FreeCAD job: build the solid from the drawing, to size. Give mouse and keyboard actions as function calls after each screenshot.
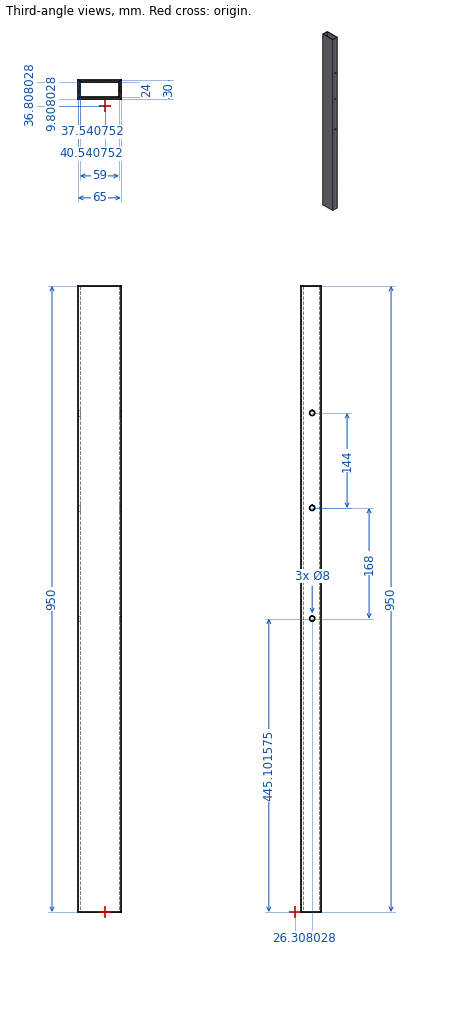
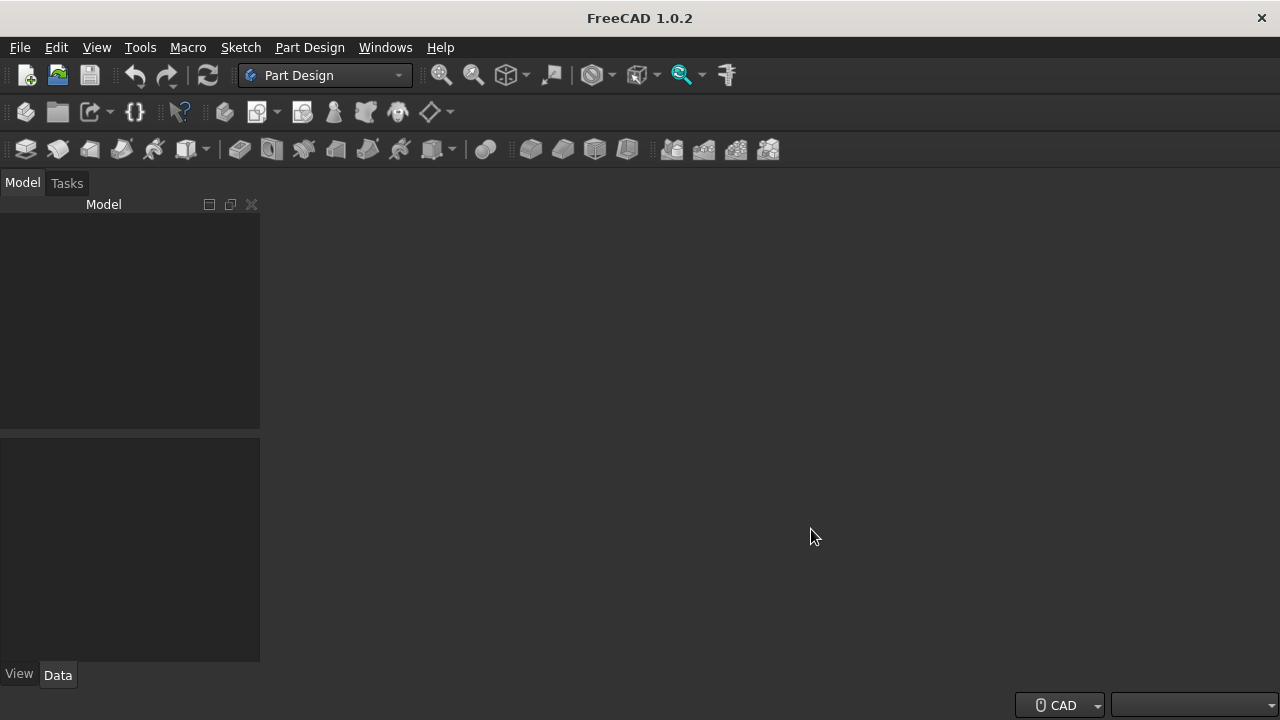
click(26, 76)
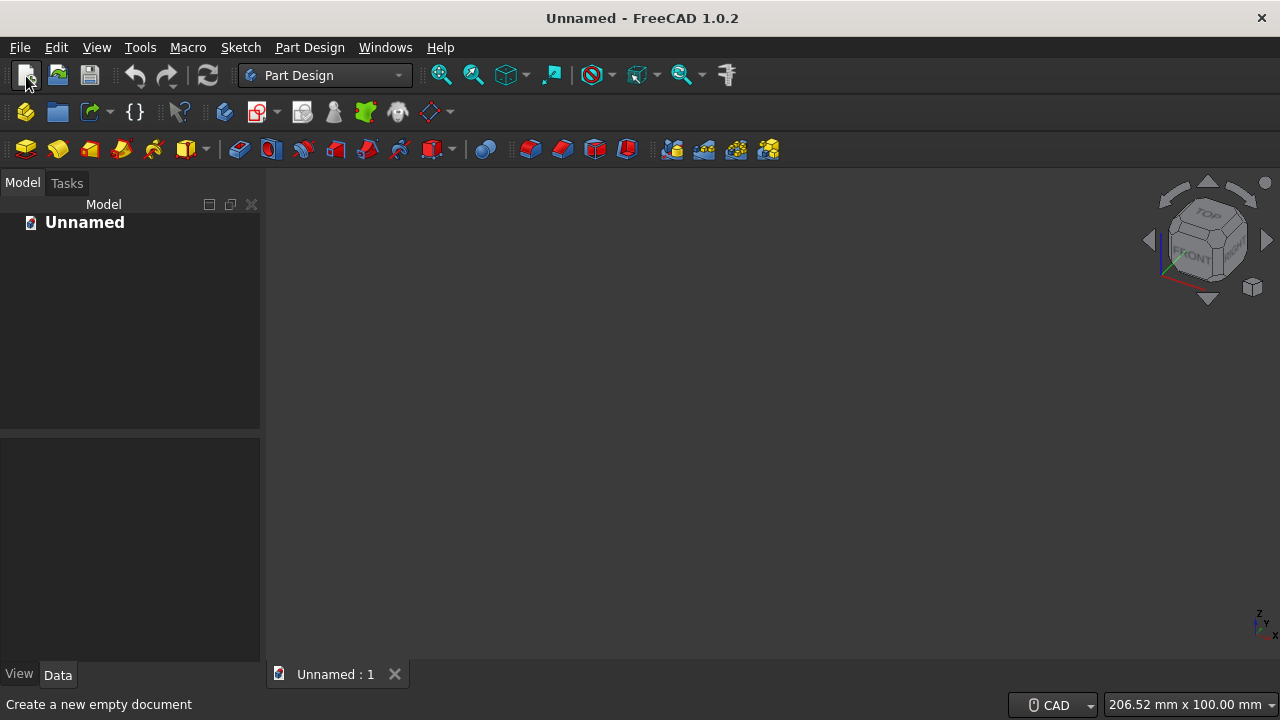
click(258, 112)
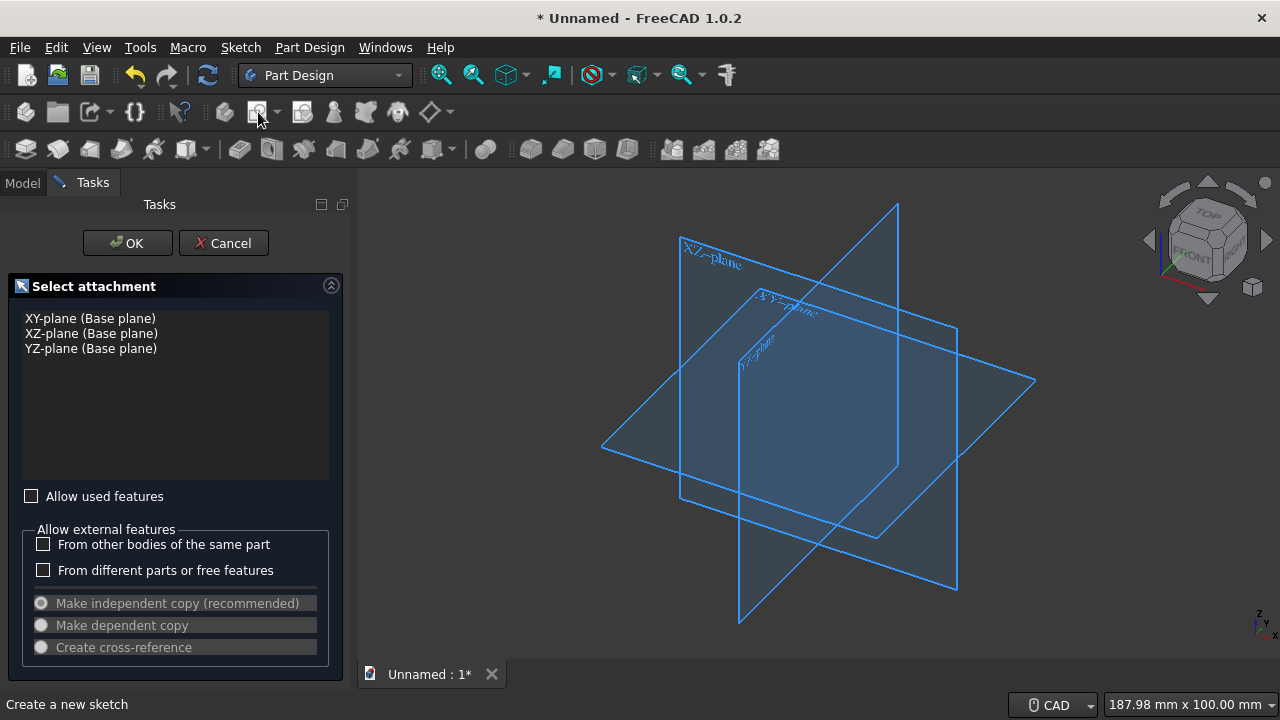
click(82, 318)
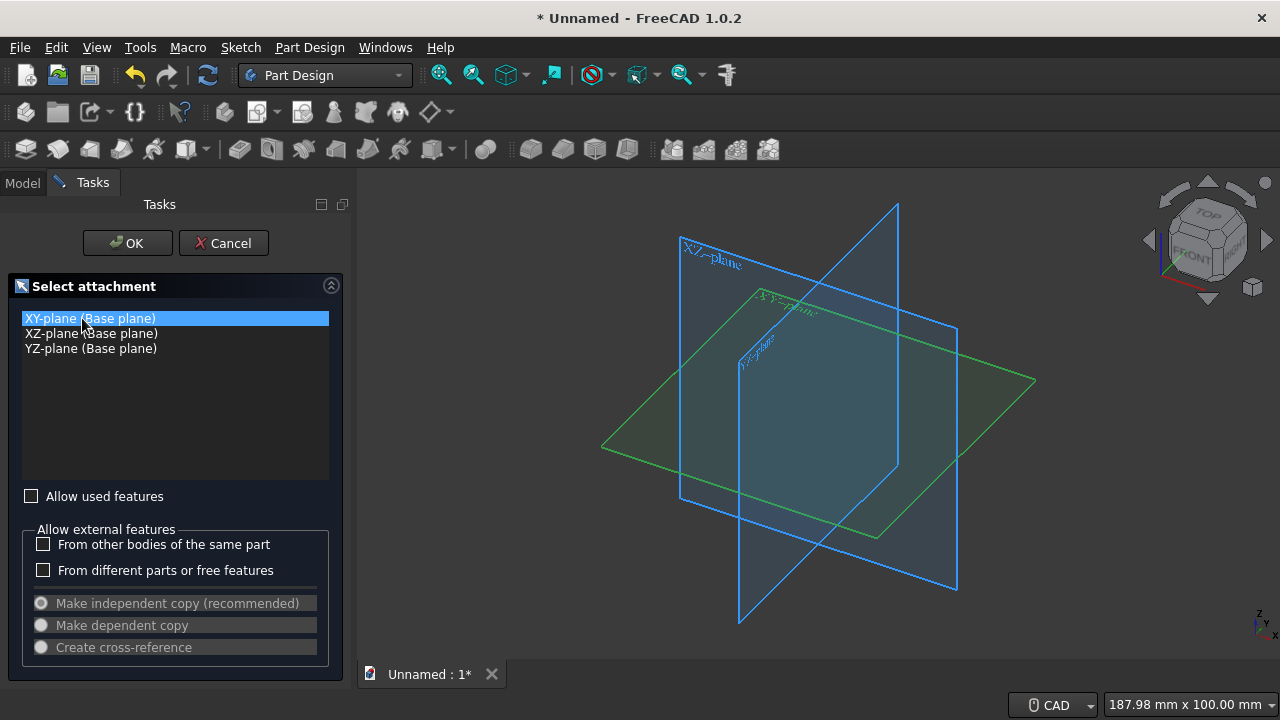
click(128, 243)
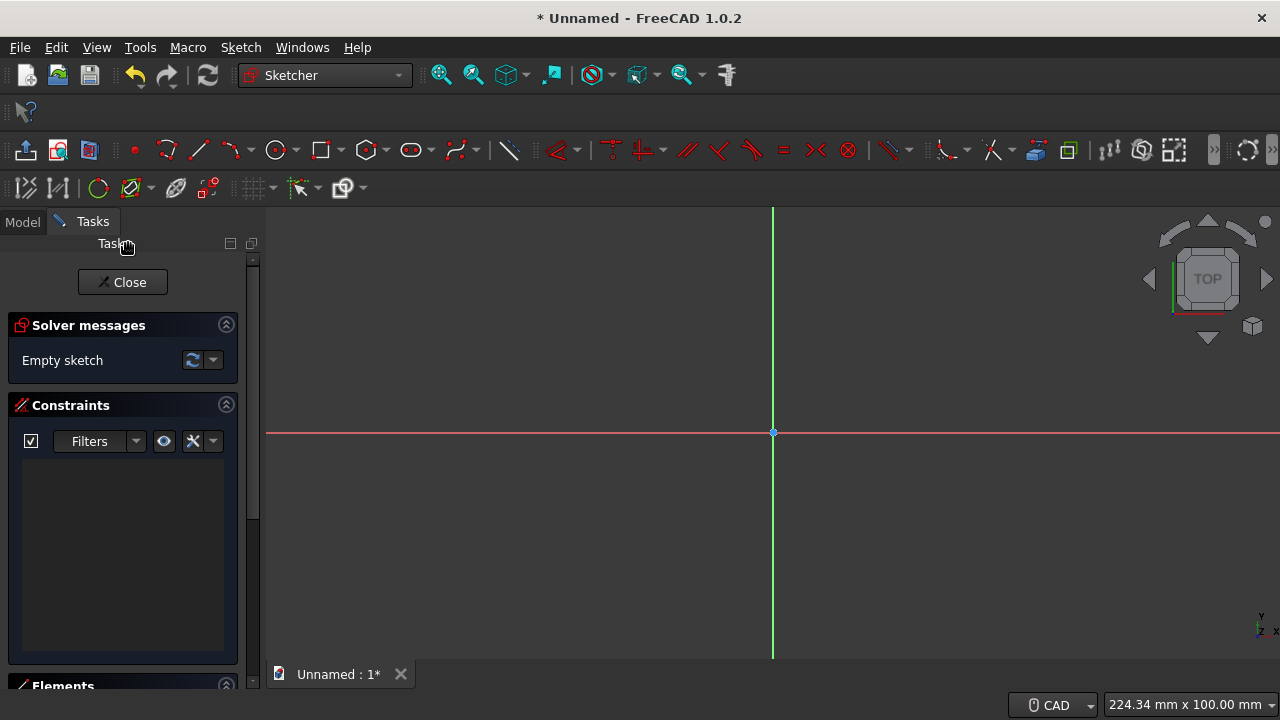
scroll(802, 235, up, 2)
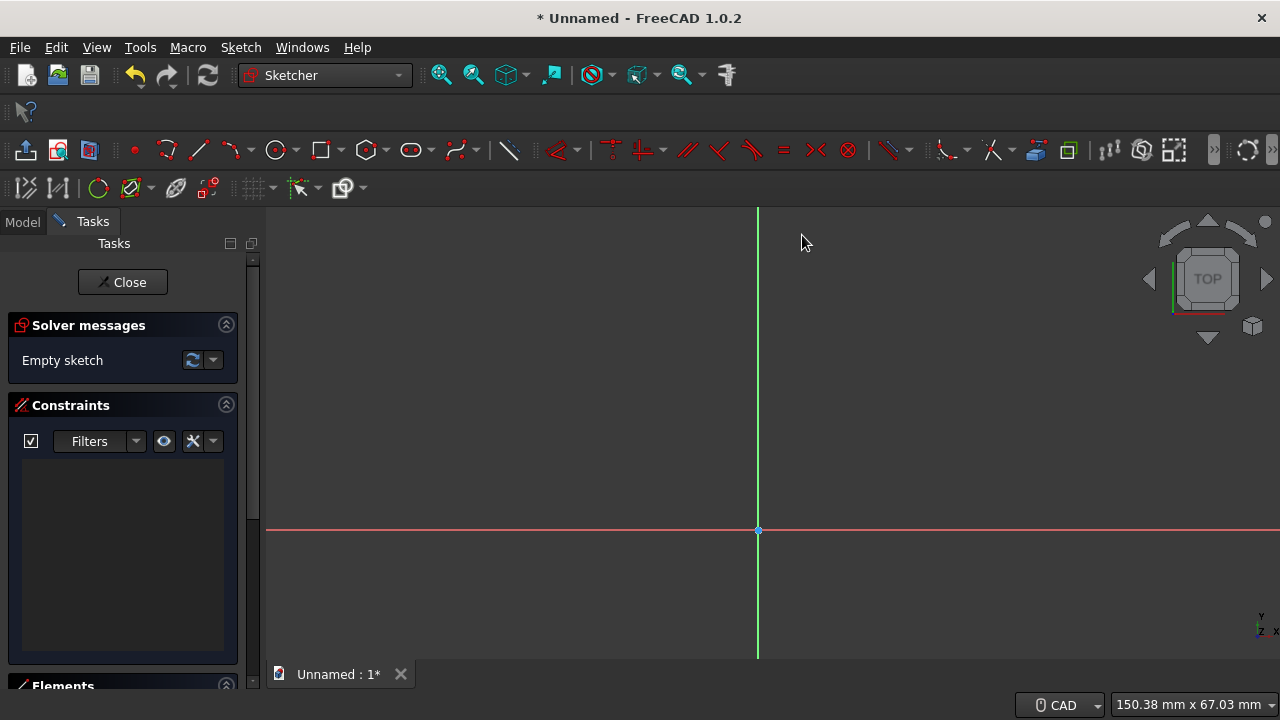
click(322, 150)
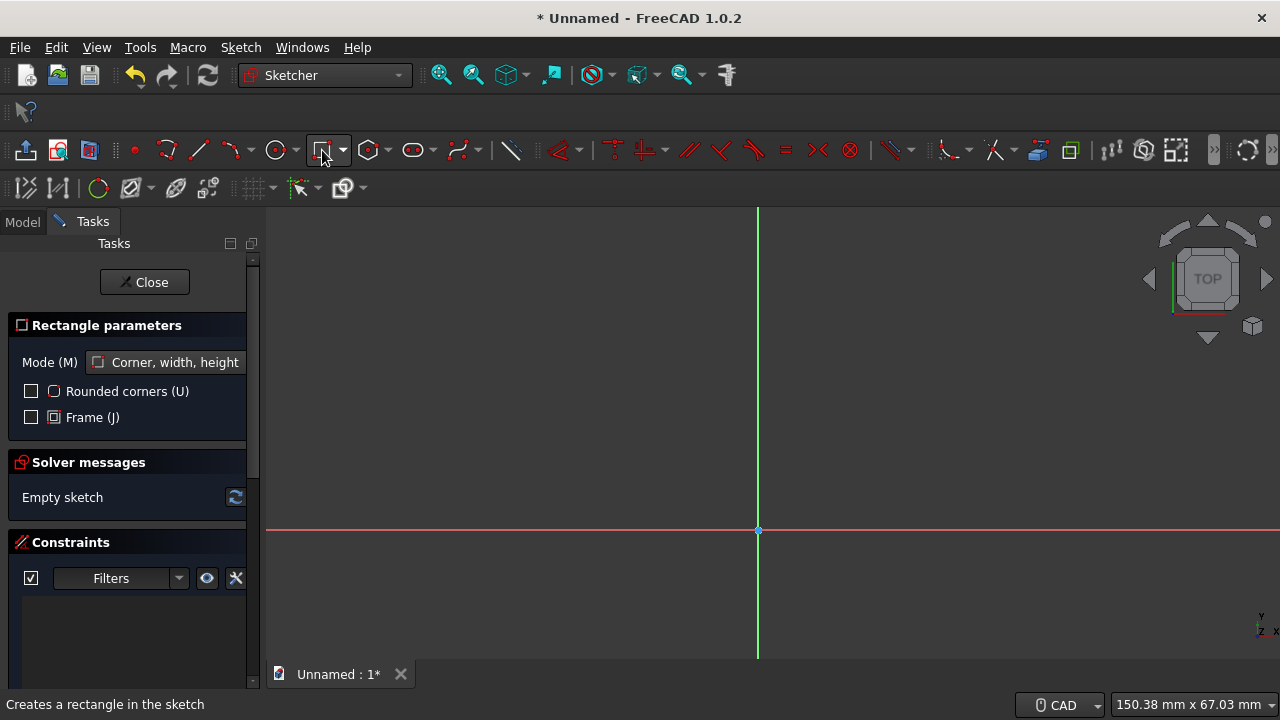
click(485, 262)
move(923, 464)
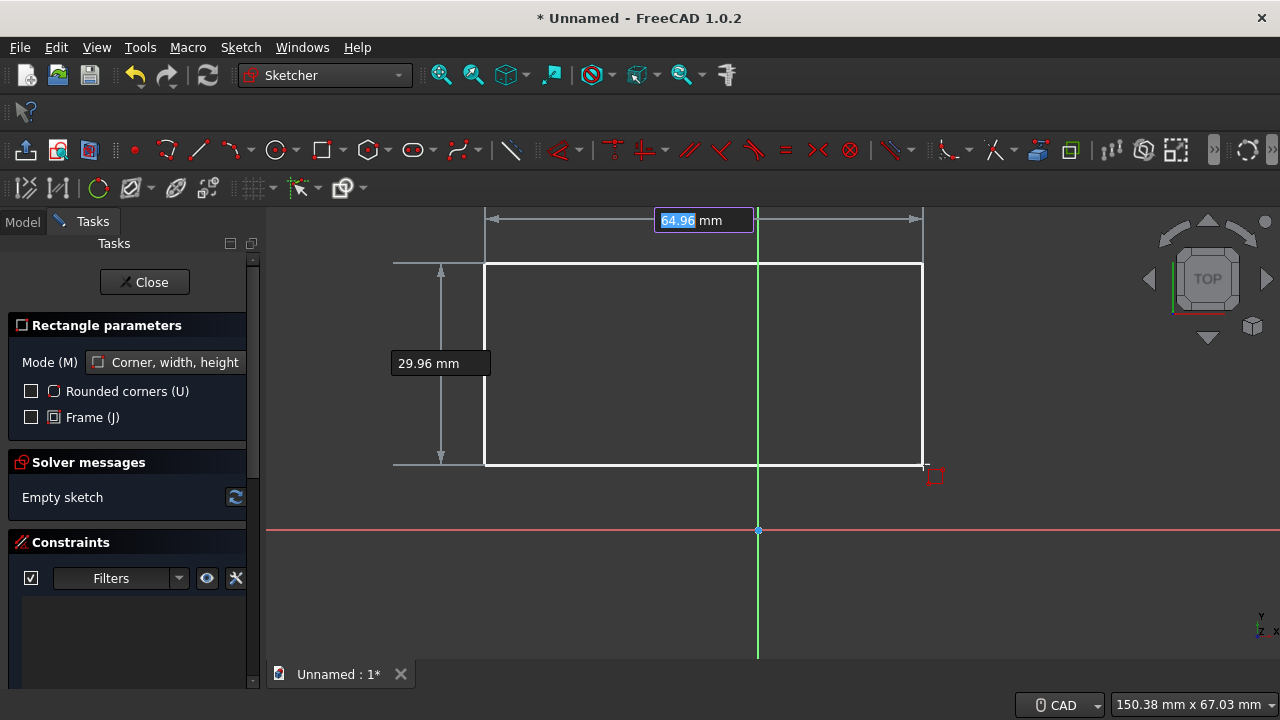
text(65)
key(Tab)
text(30)
key(Return)
key(Escape)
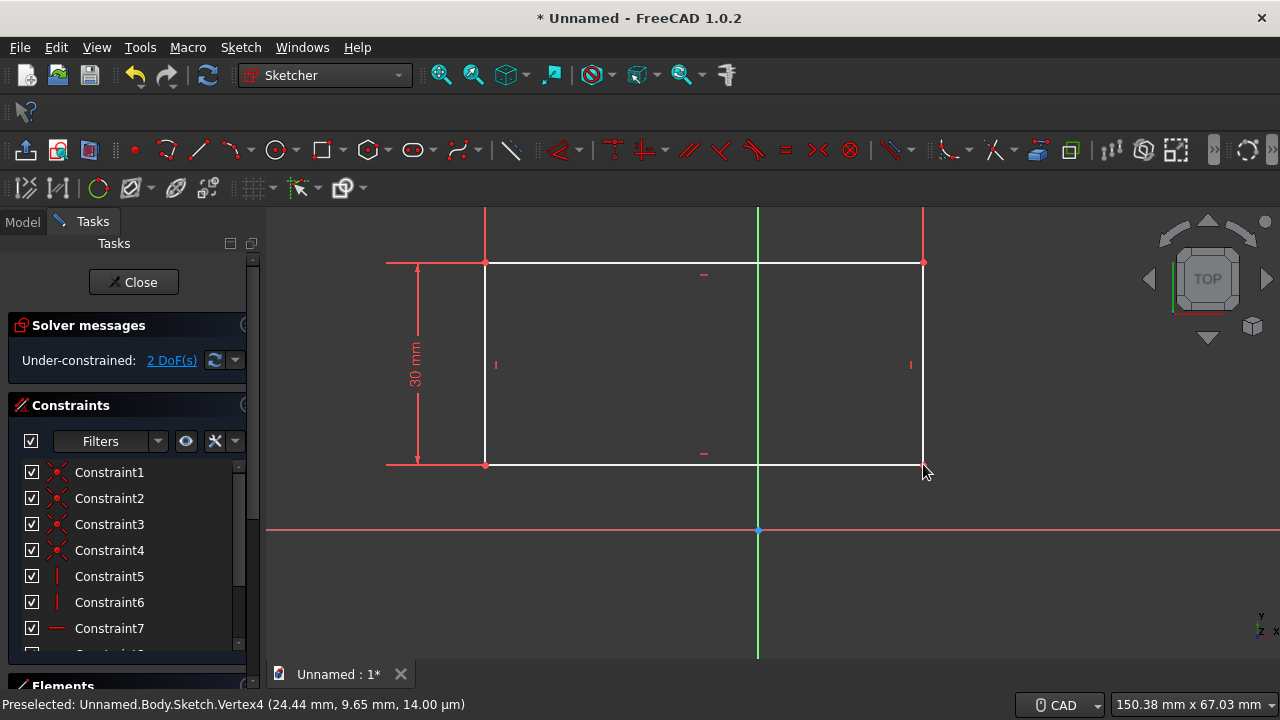
click(558, 150)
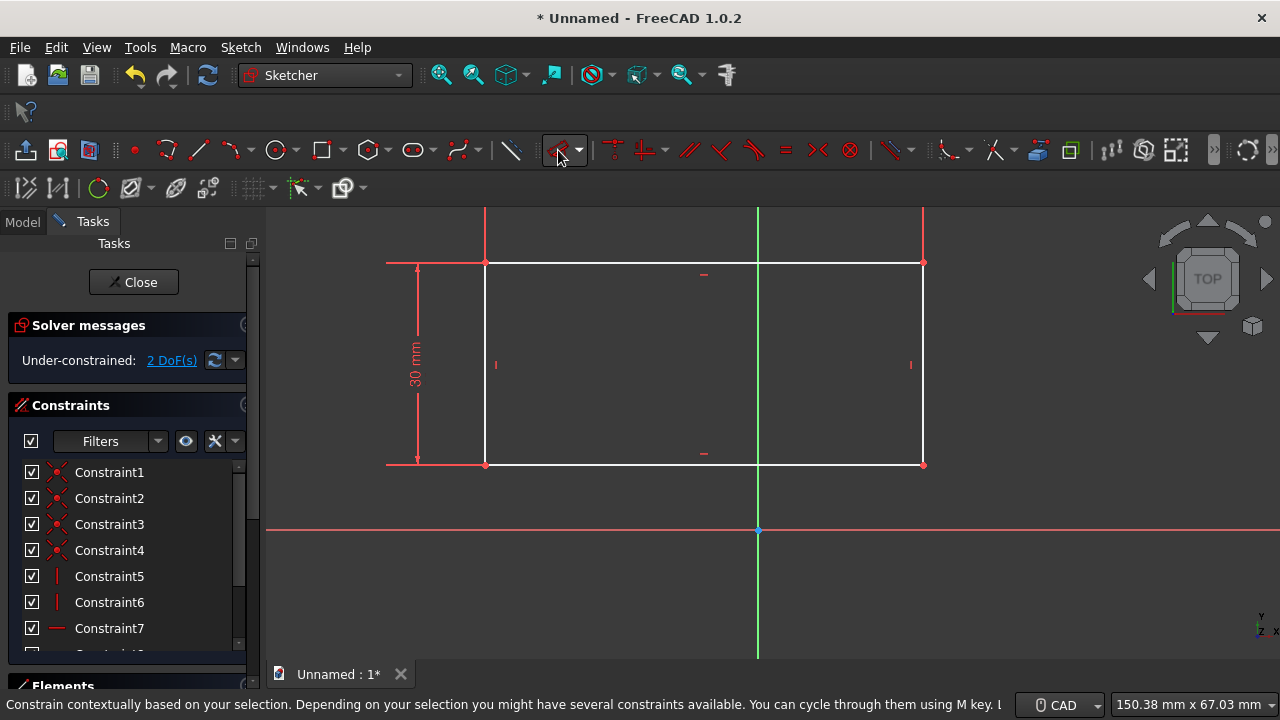
click(485, 465)
click(451, 498)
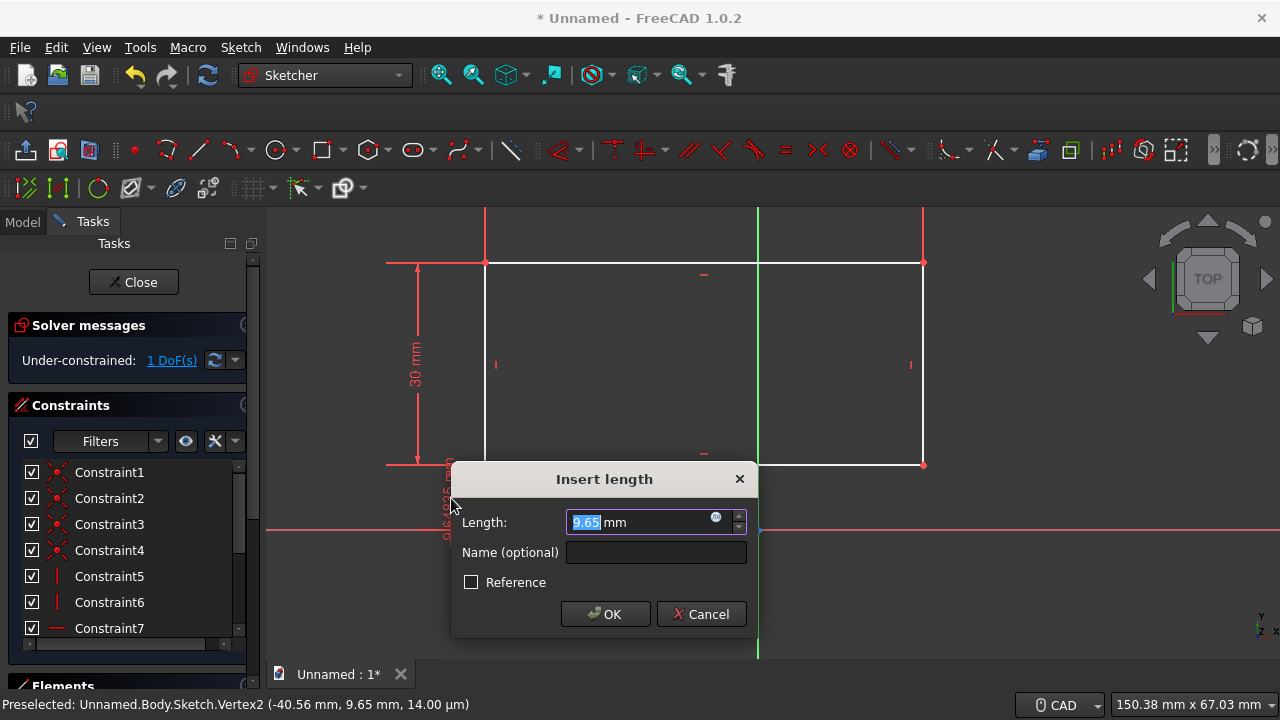
text(9.808028)
key(Return)